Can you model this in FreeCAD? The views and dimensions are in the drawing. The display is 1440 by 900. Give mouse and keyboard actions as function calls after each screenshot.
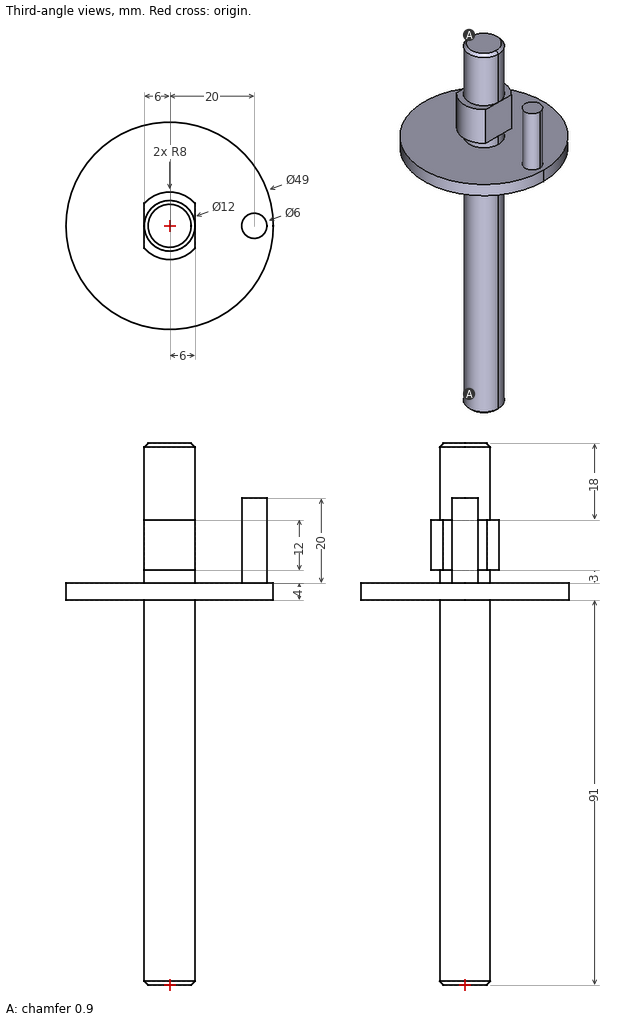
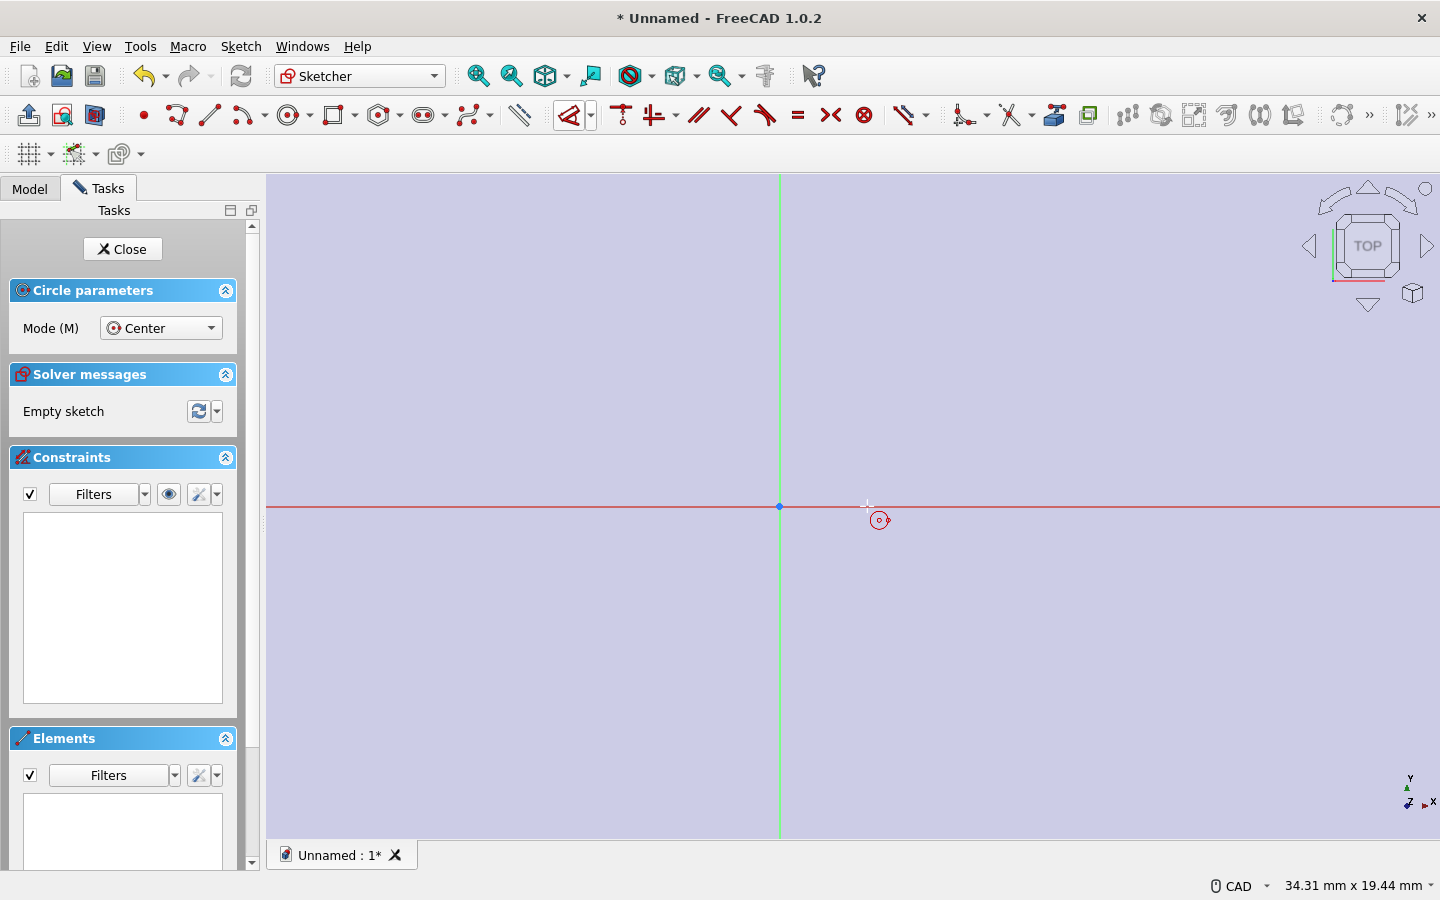
click(780, 506)
click(925, 361)
key(Escape)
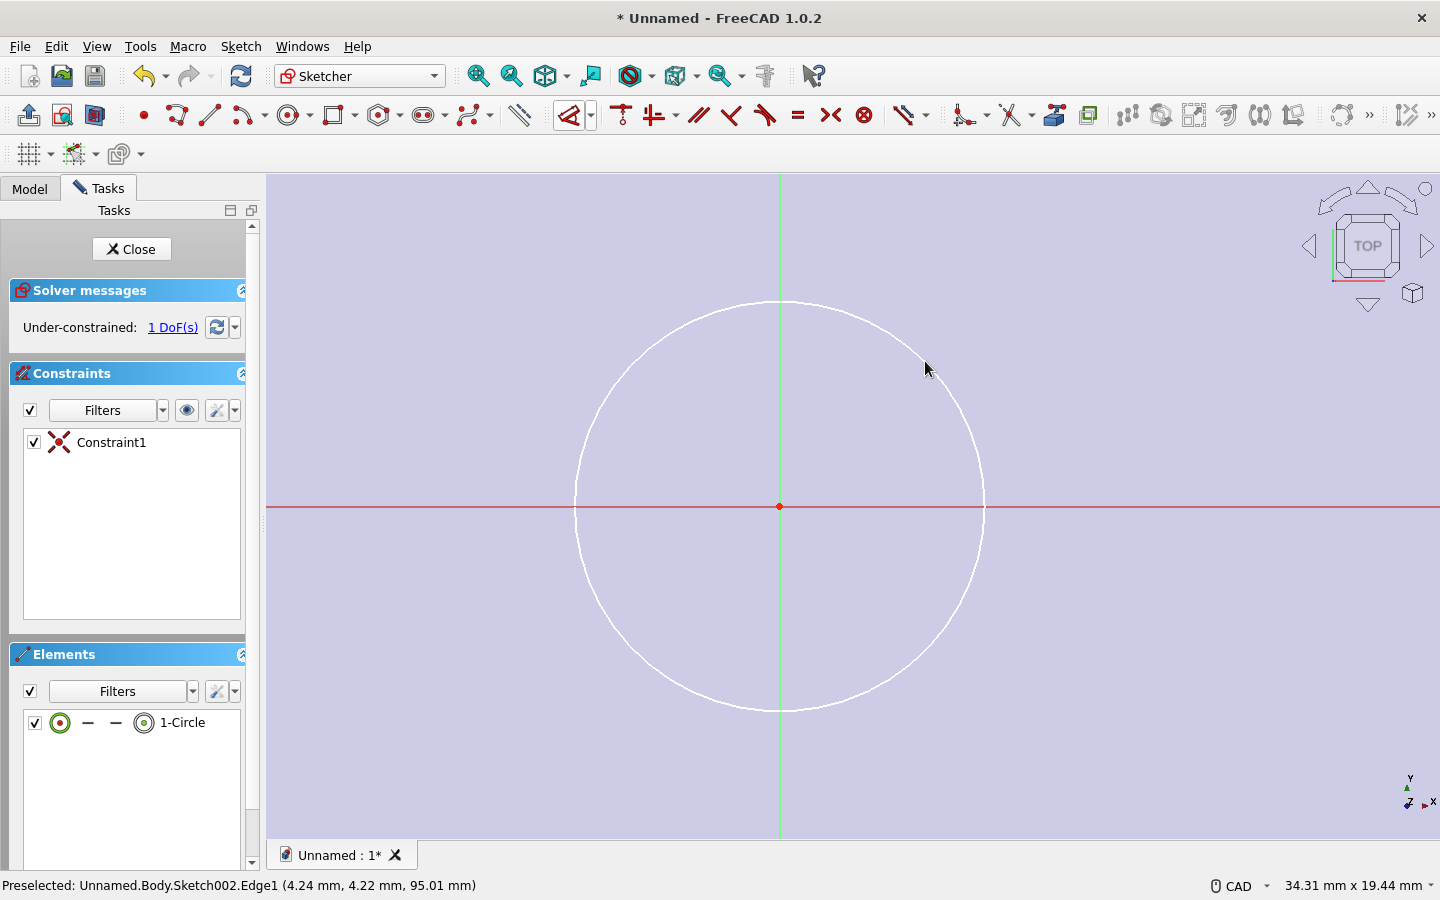
click(924, 361)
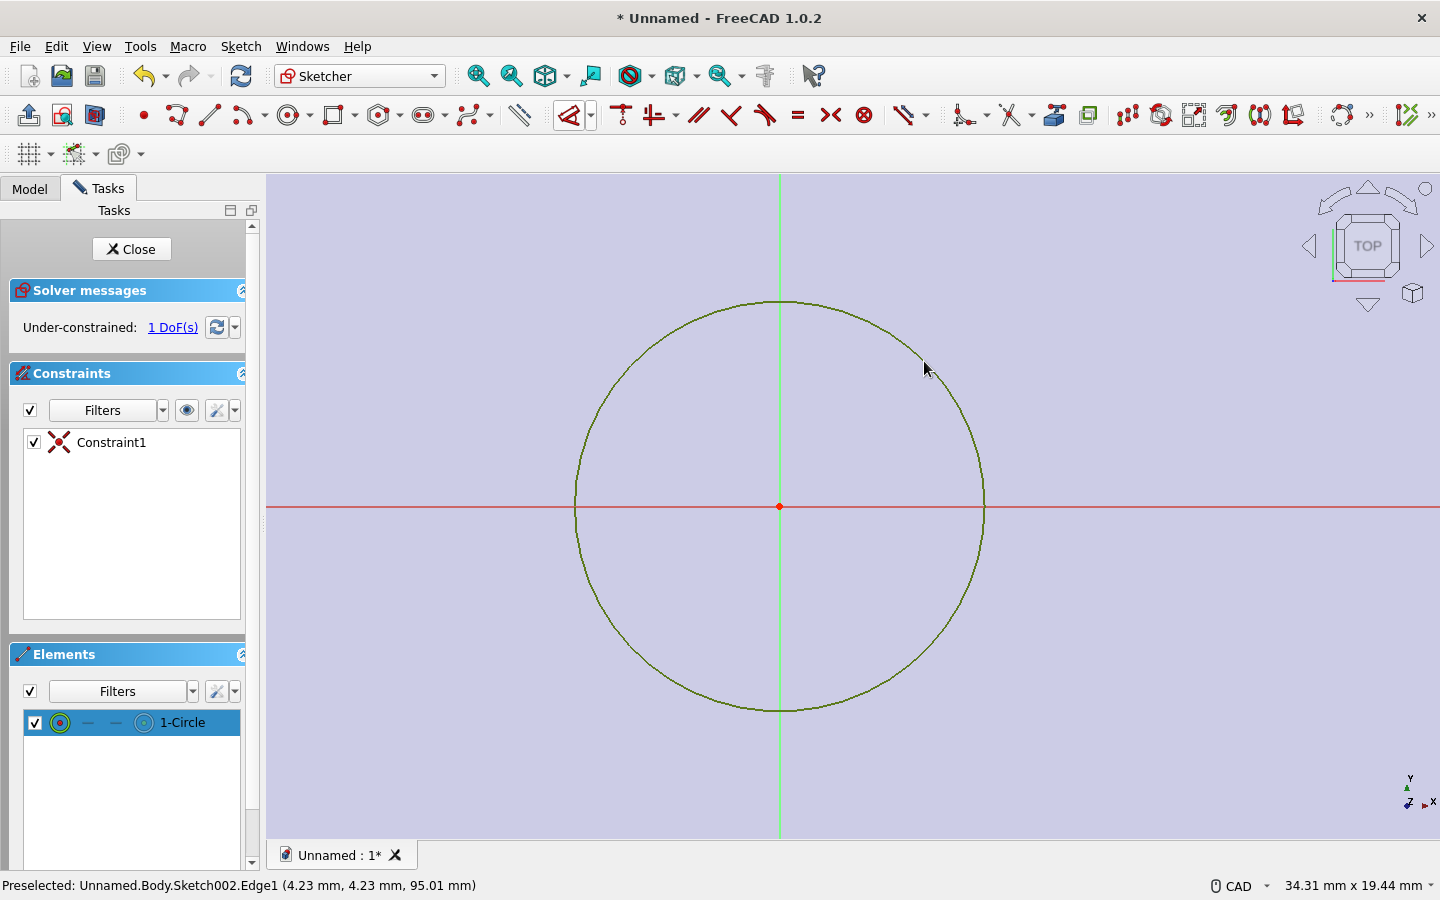
click(590, 116)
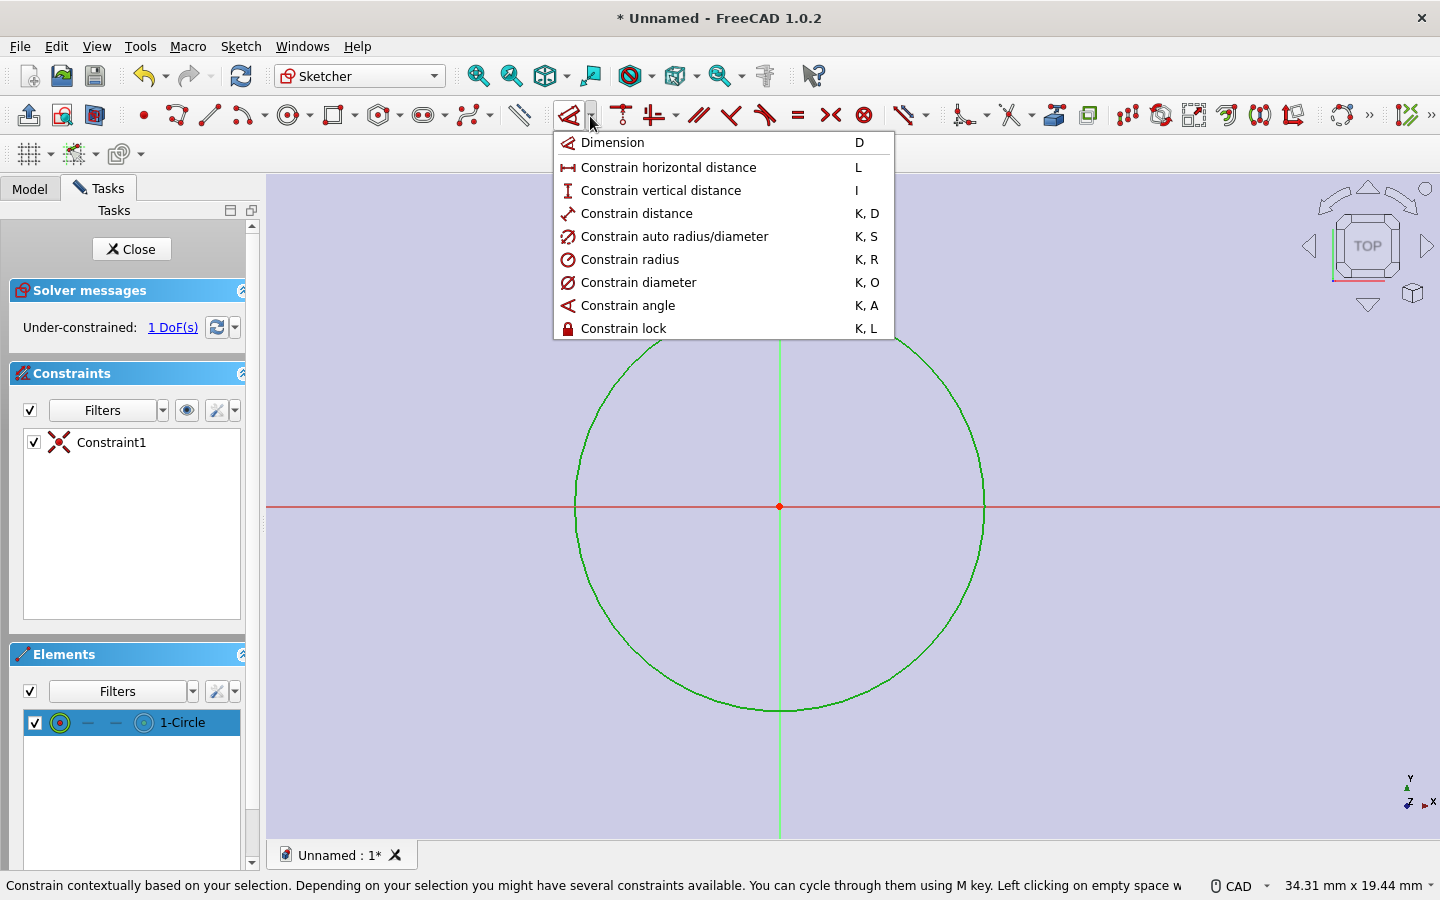
click(724, 282)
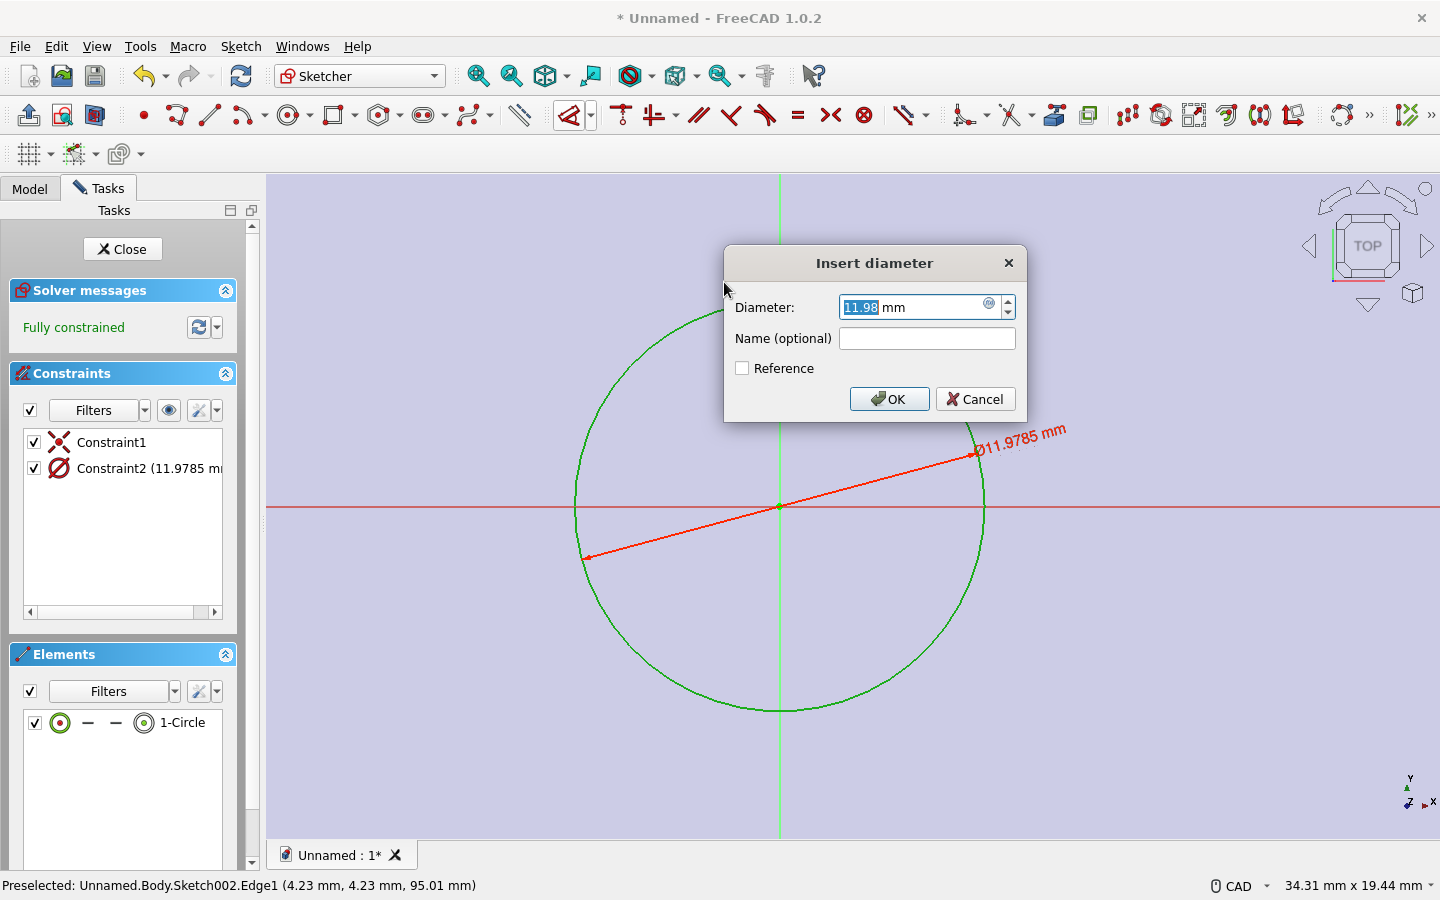
text(12)
key(Return)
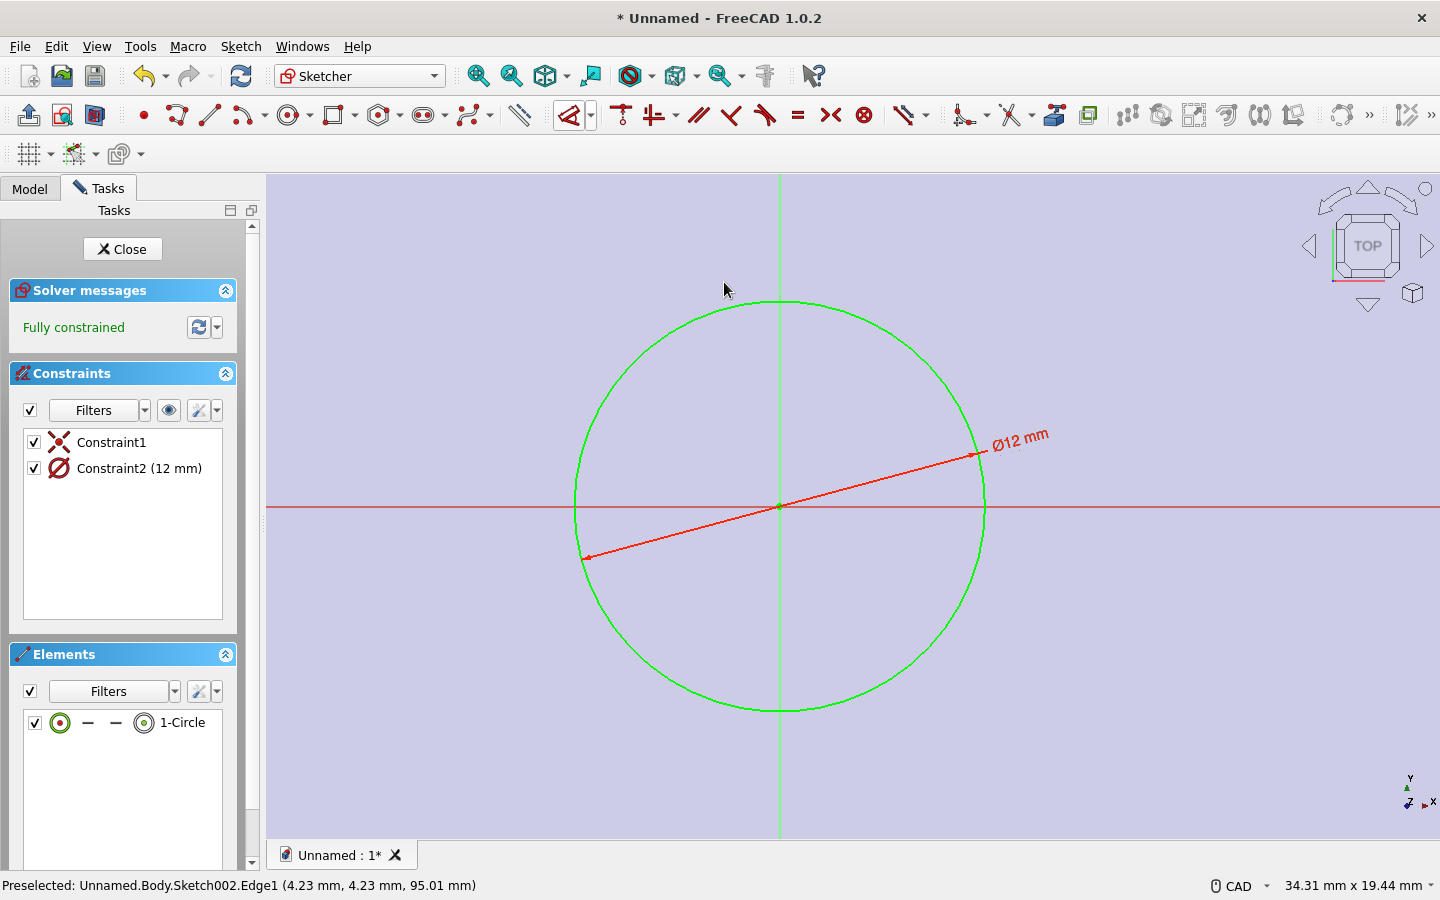
click(123, 249)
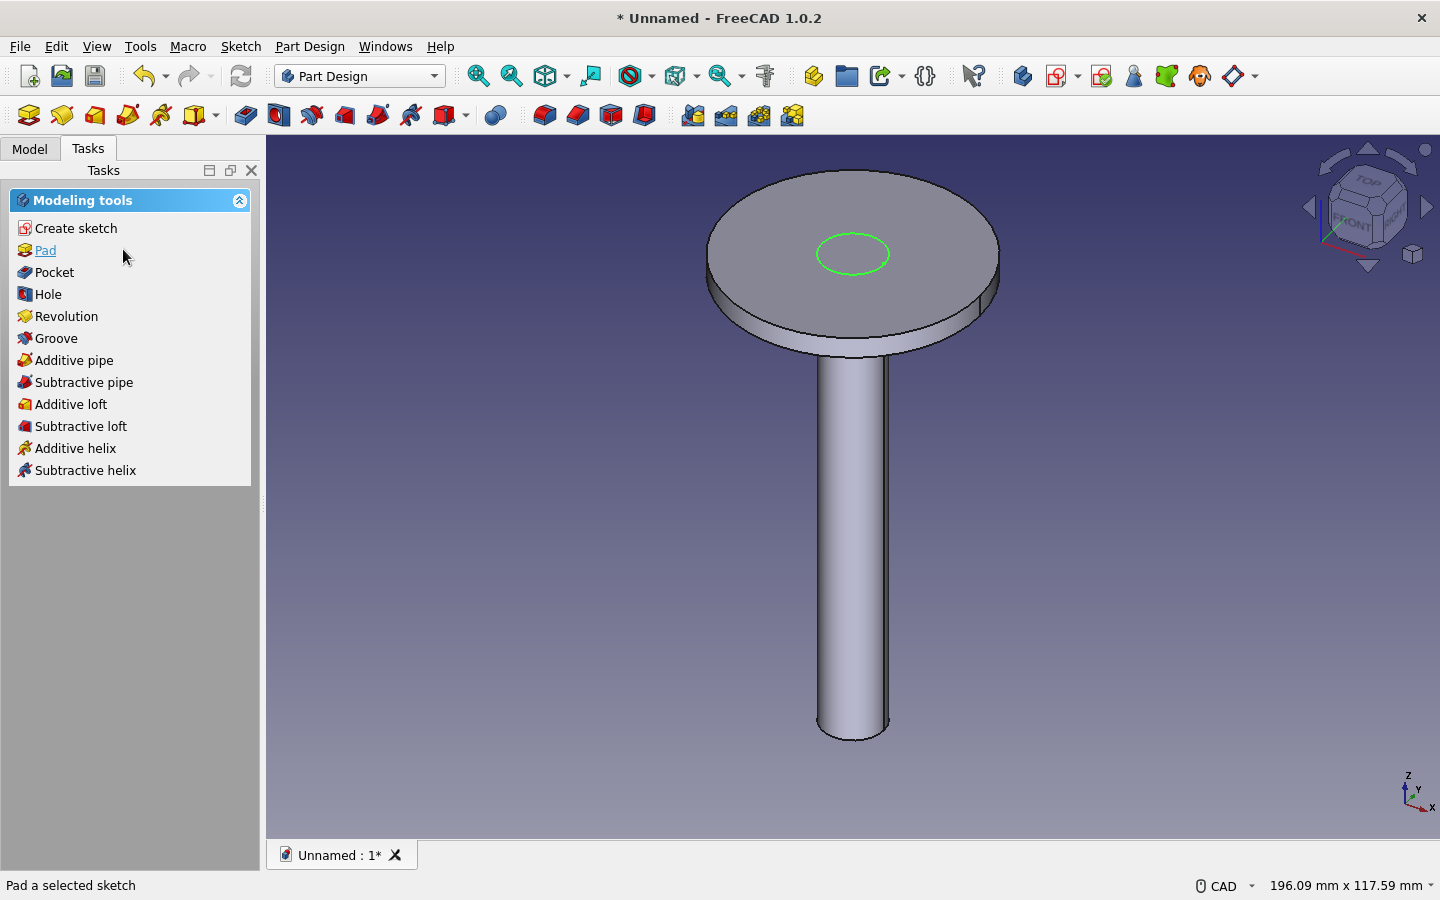
click(29, 116)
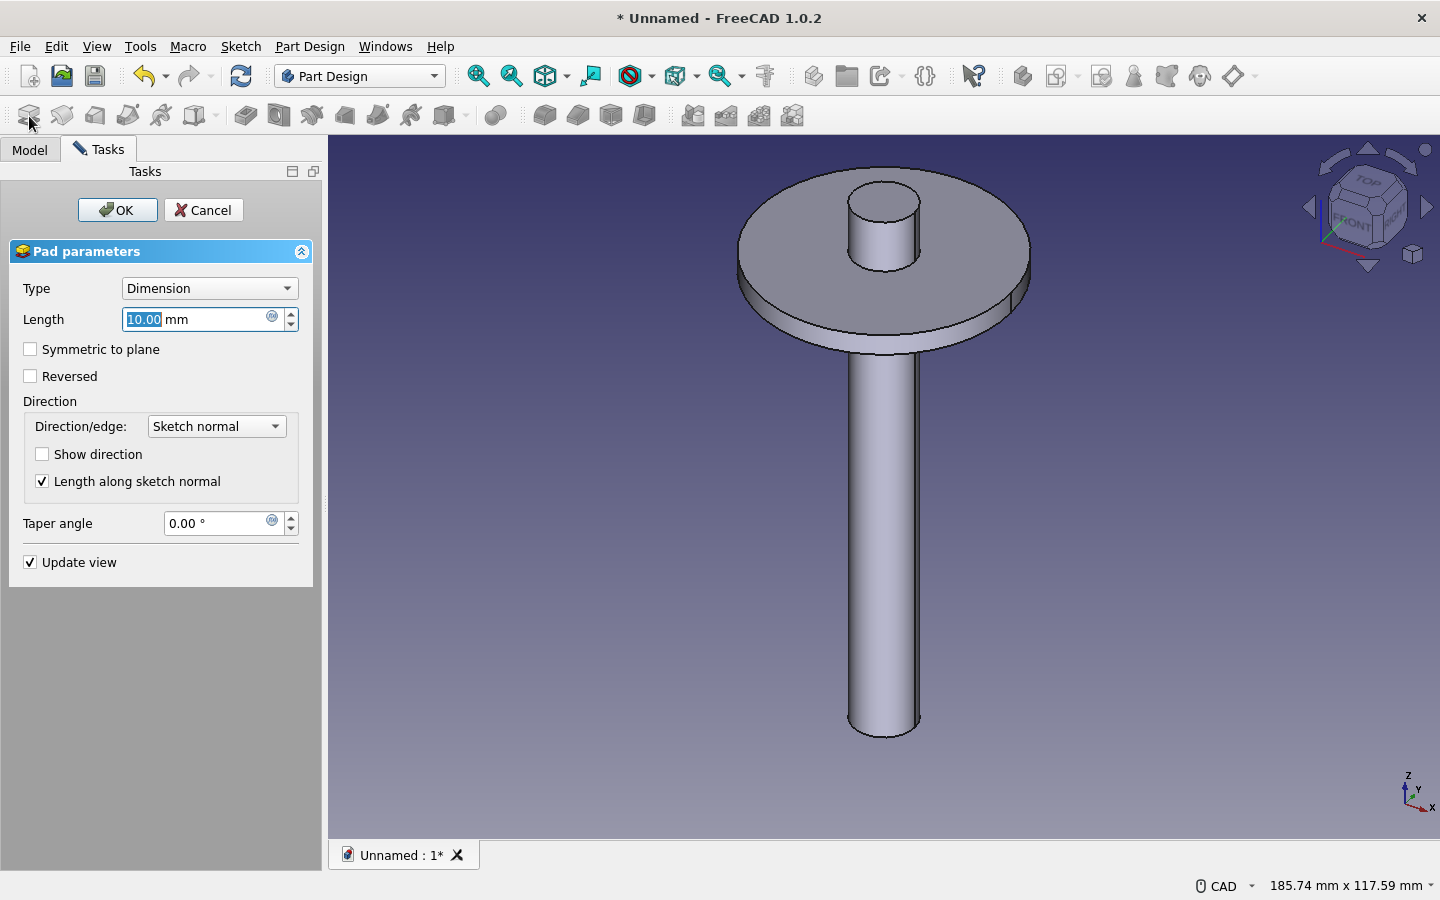
text(3)
key(Tab)